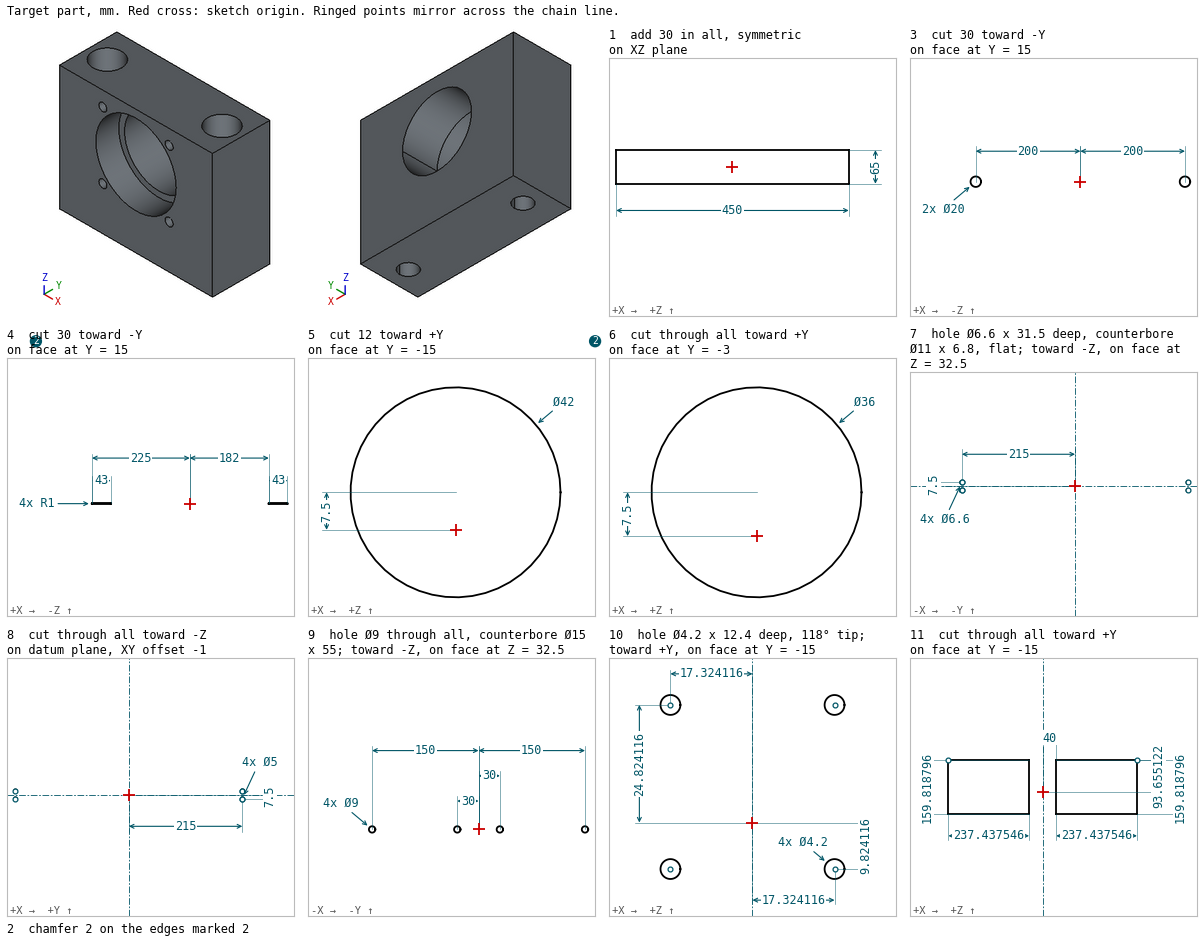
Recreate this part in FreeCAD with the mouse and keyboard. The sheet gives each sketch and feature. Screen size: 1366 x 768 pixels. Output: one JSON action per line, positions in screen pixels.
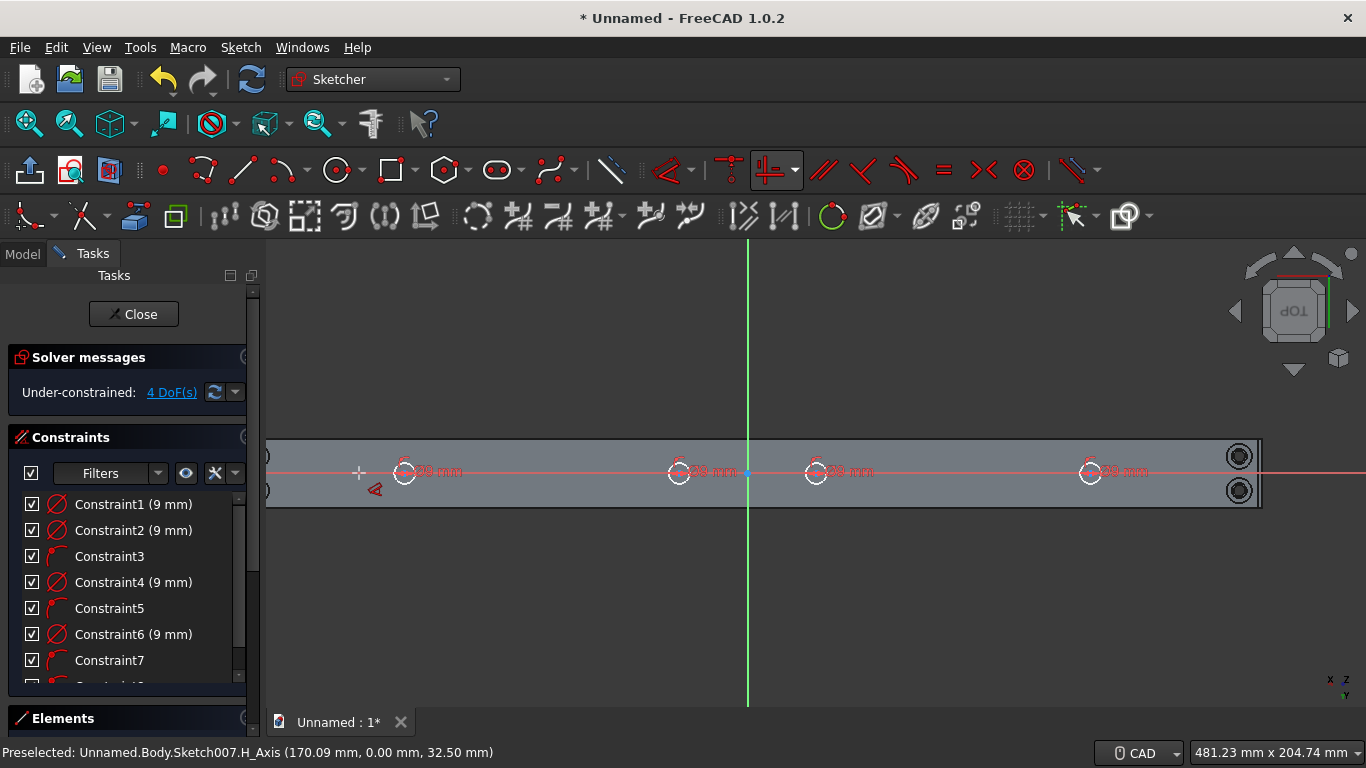
{"action": "left_click", "coordinate": [679, 473]}
{"action": "left_click", "coordinate": [714, 507]}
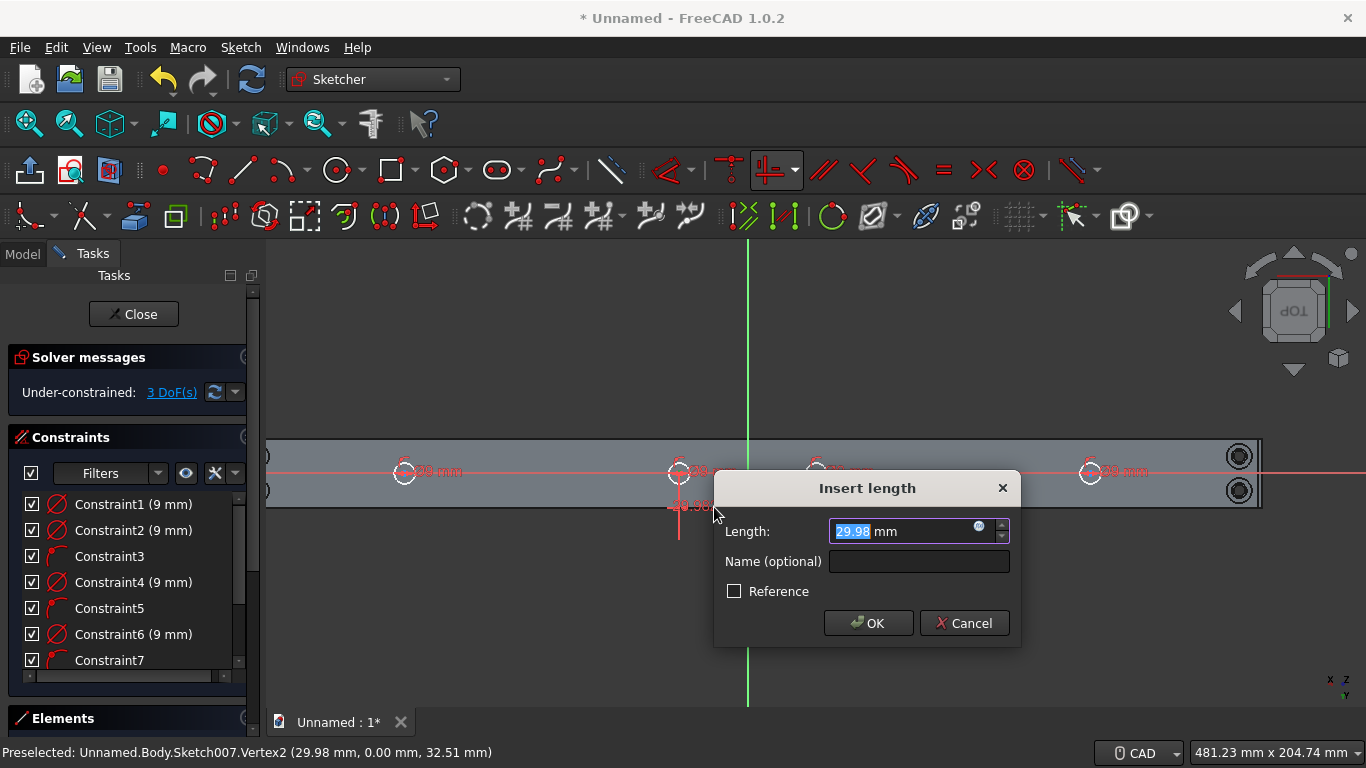
{"action": "type", "text": "30"}
{"action": "key", "text": "Return"}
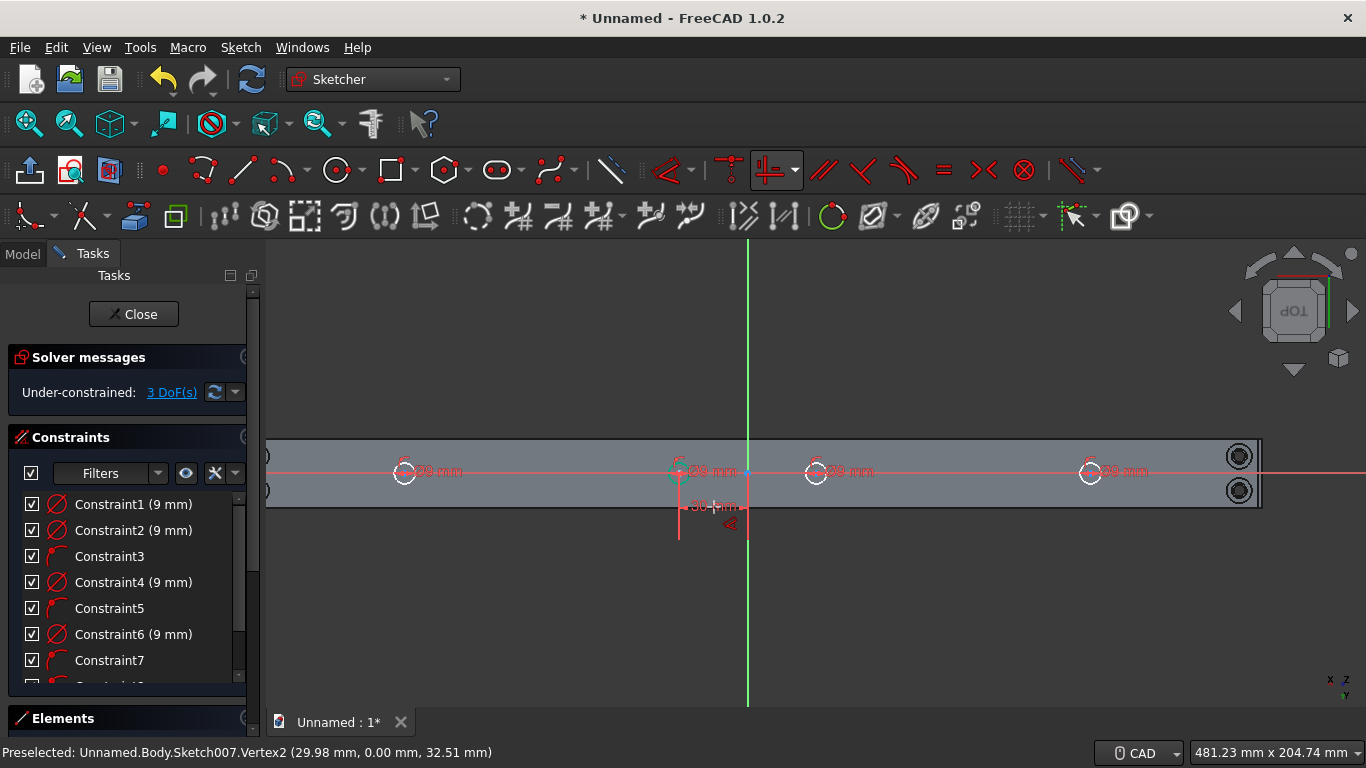
{"action": "left_click", "coordinate": [816, 473]}
{"action": "left_click", "coordinate": [798, 507]}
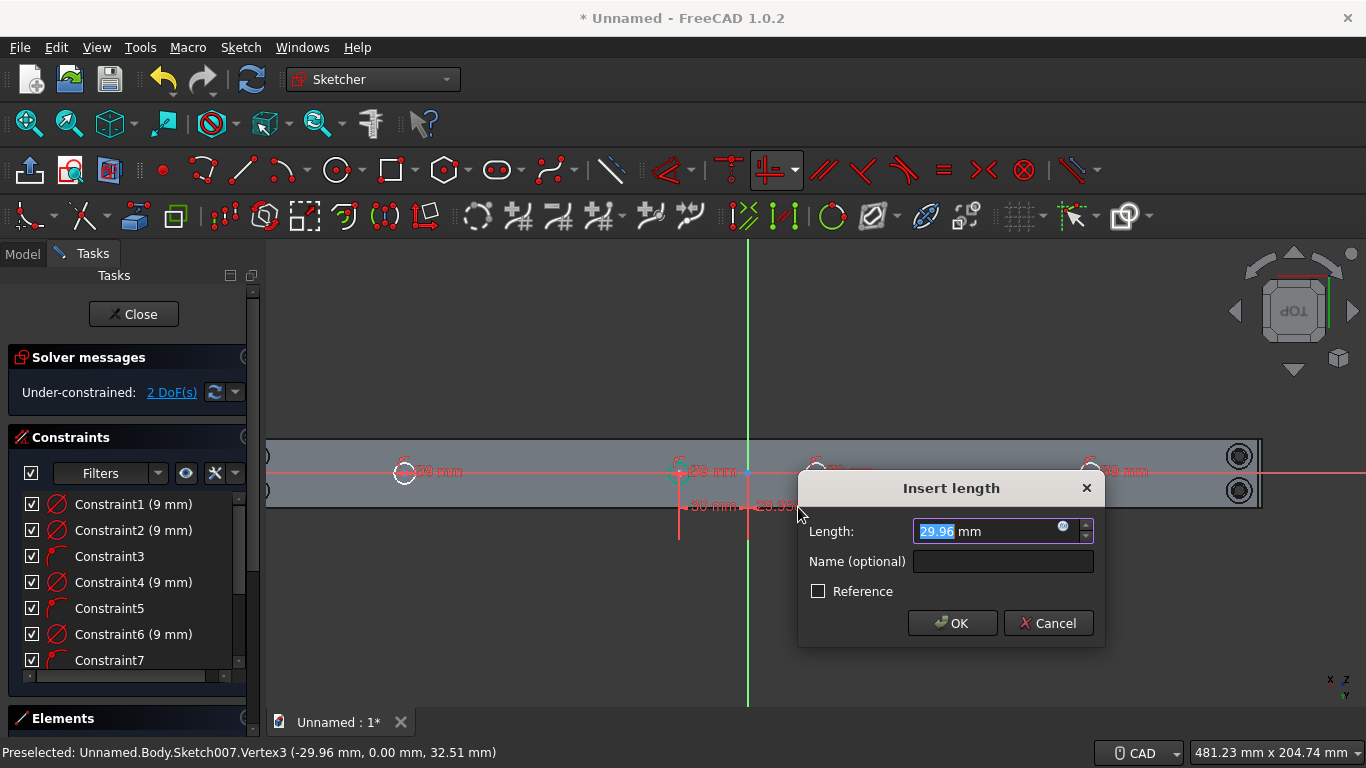
{"action": "type", "text": "30"}
{"action": "key", "text": "Return"}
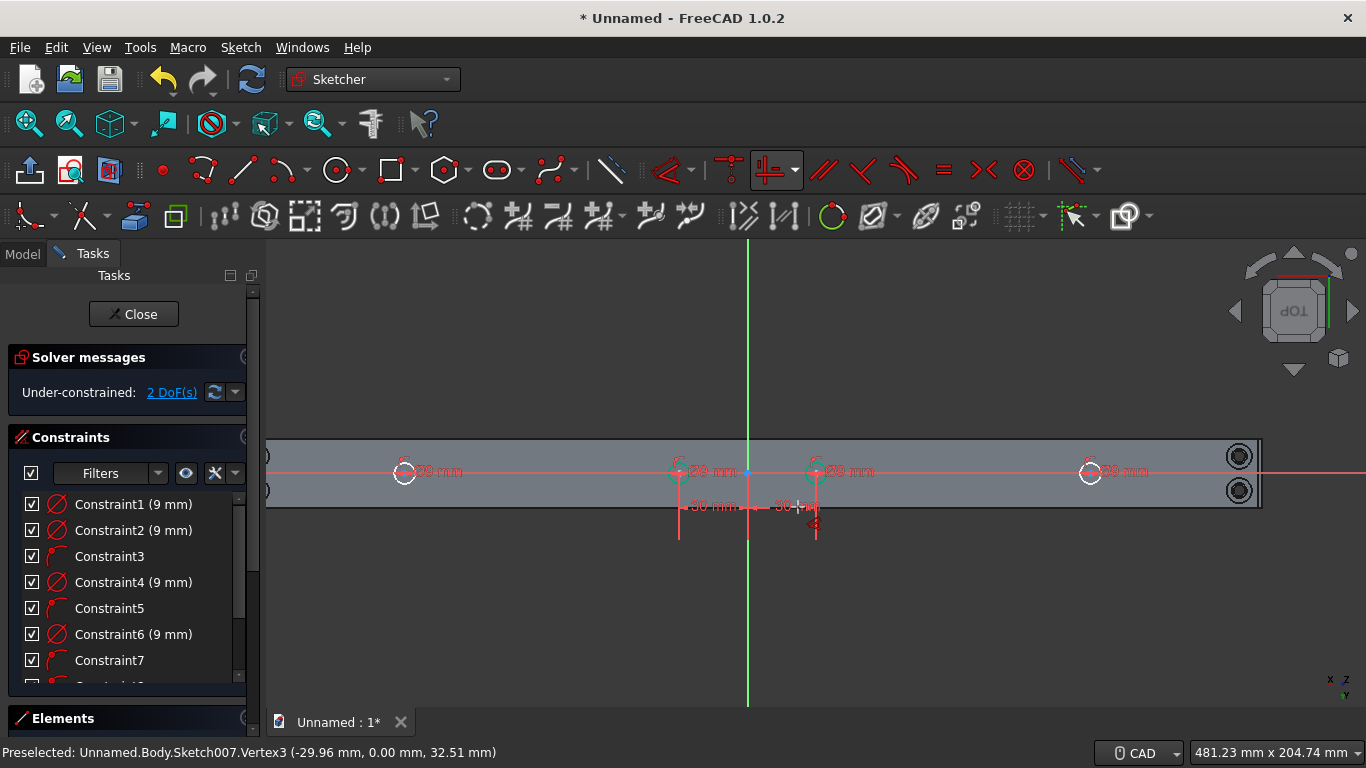
{"action": "left_click", "coordinate": [405, 473]}
{"action": "left_click", "coordinate": [576, 507]}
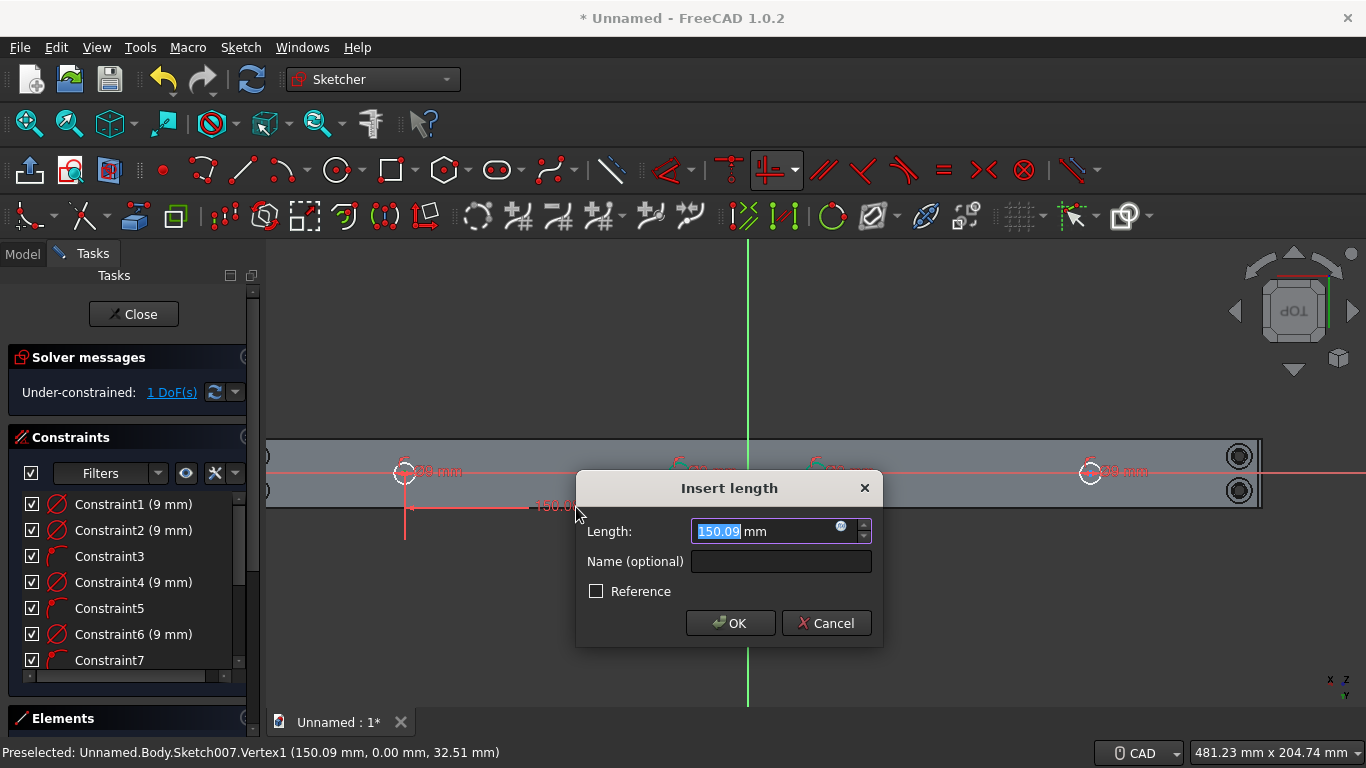
{"action": "type", "text": "150"}
{"action": "key", "text": "Return"}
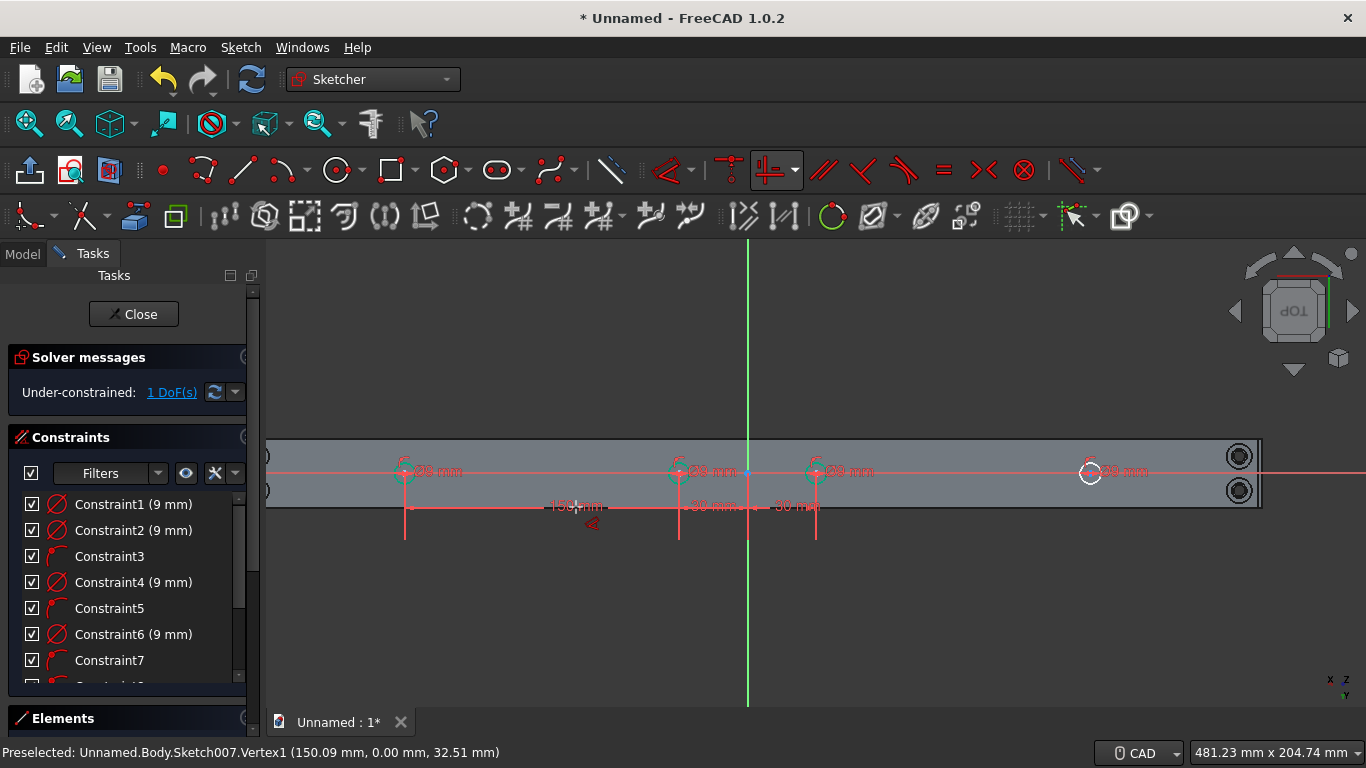
{"action": "left_click", "coordinate": [1091, 473]}
{"action": "left_click", "coordinate": [919, 507]}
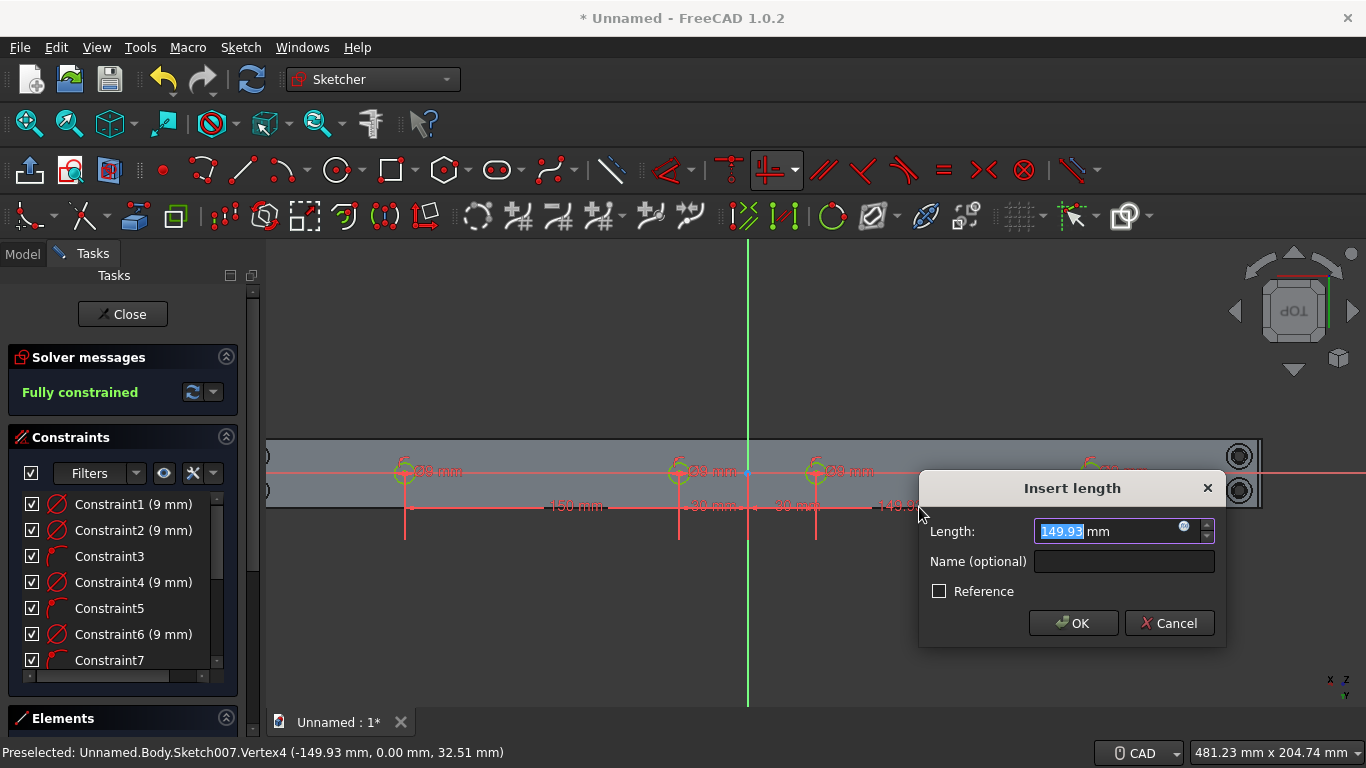
{"action": "type", "text": "150"}
{"action": "key", "text": "Return"}
{"action": "key", "text": "Escape"}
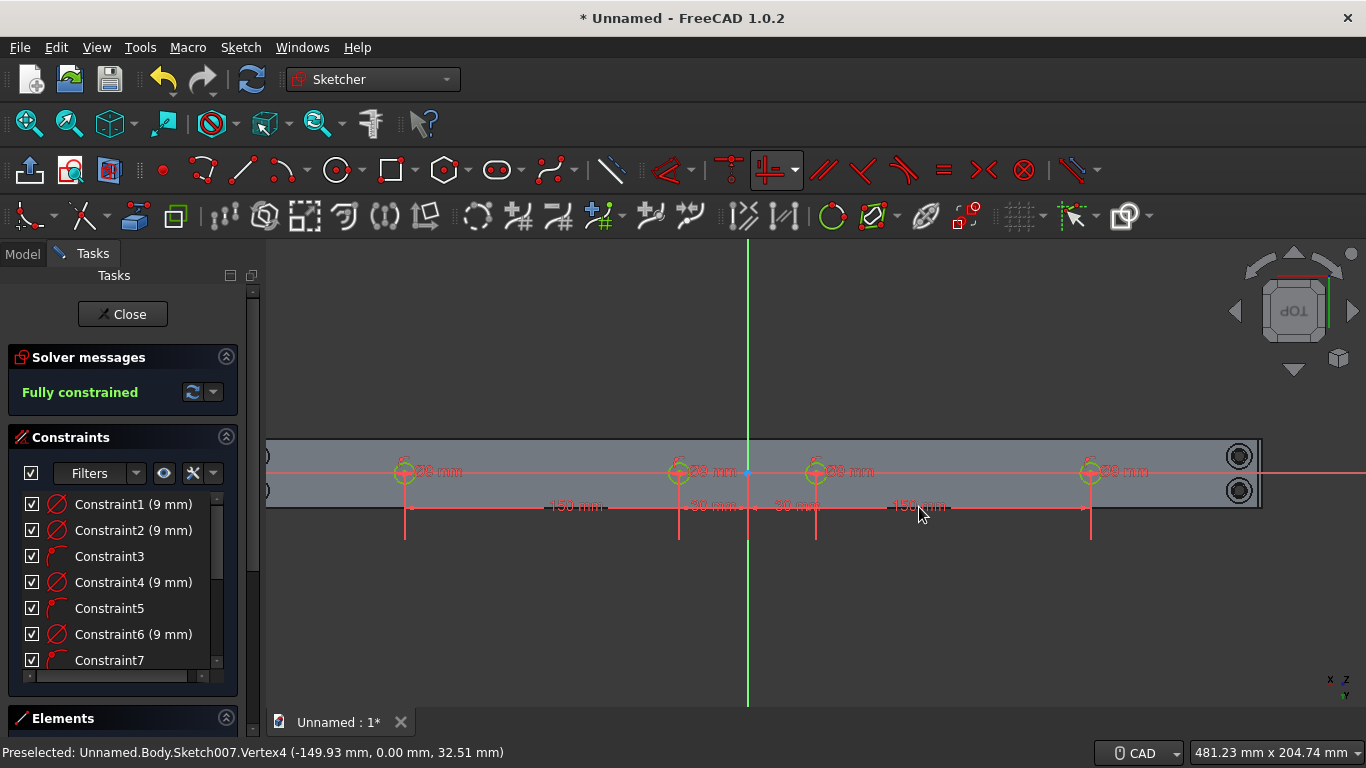
{"action": "left_click", "coordinate": [123, 314]}